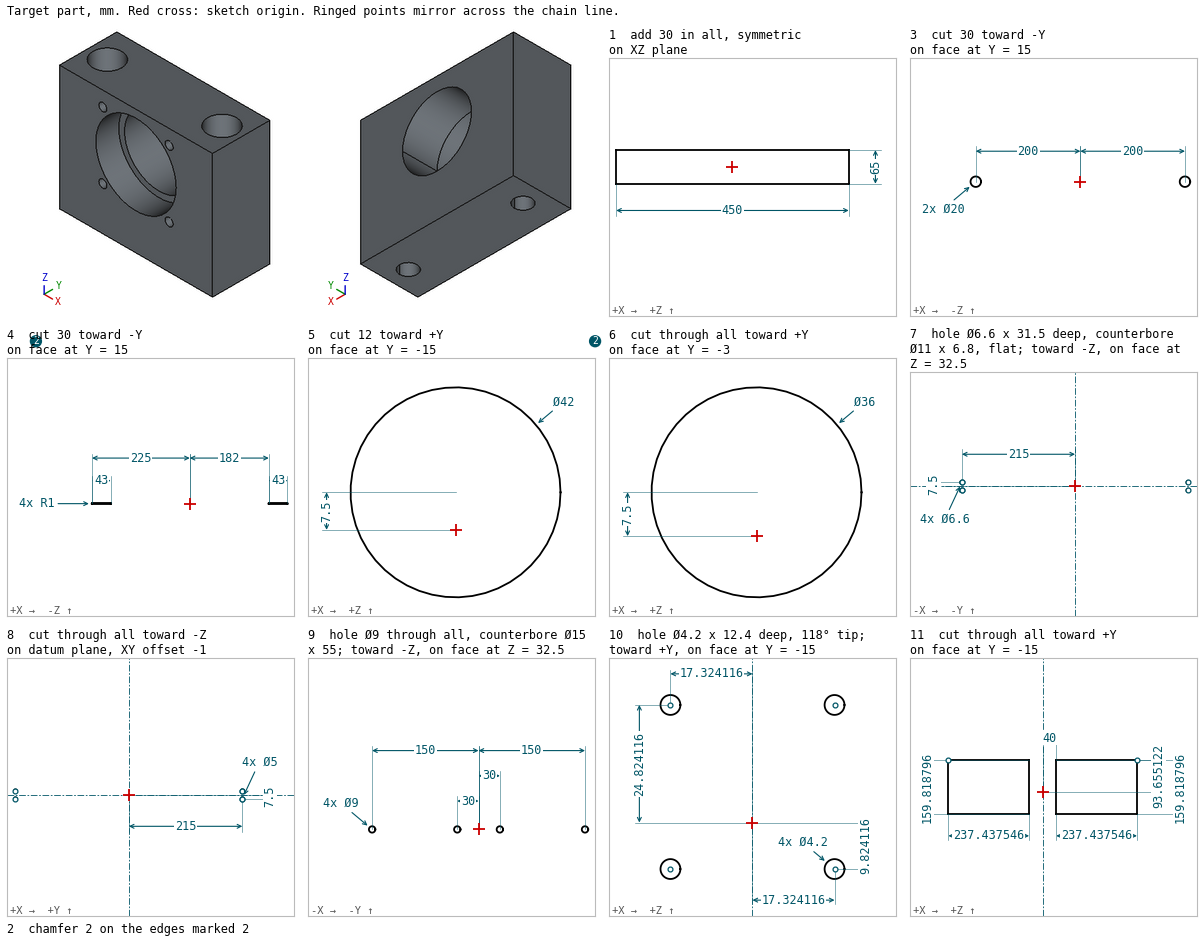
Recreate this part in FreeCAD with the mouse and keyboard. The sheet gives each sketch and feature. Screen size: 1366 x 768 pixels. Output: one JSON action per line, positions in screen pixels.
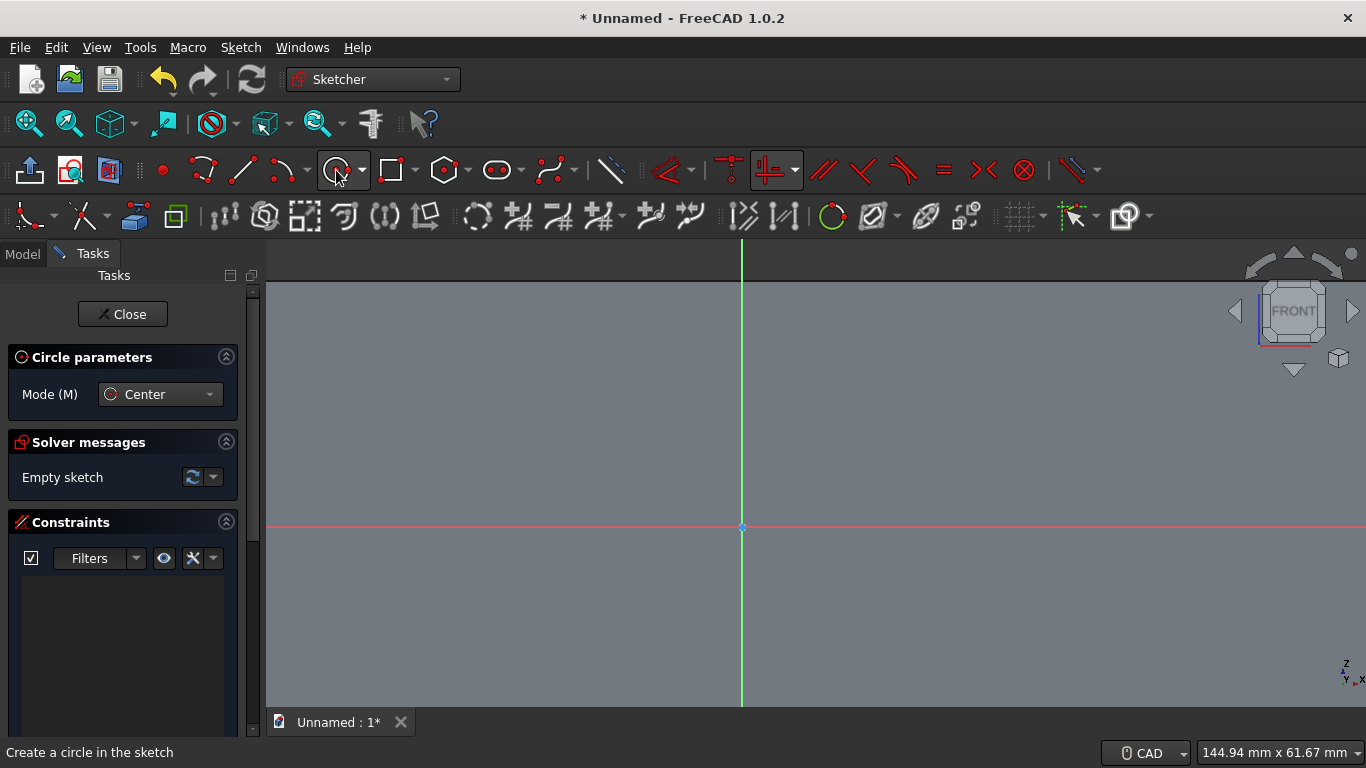
{"action": "left_click", "coordinate": [742, 471]}
{"action": "mouse_move", "coordinate": [855, 358]}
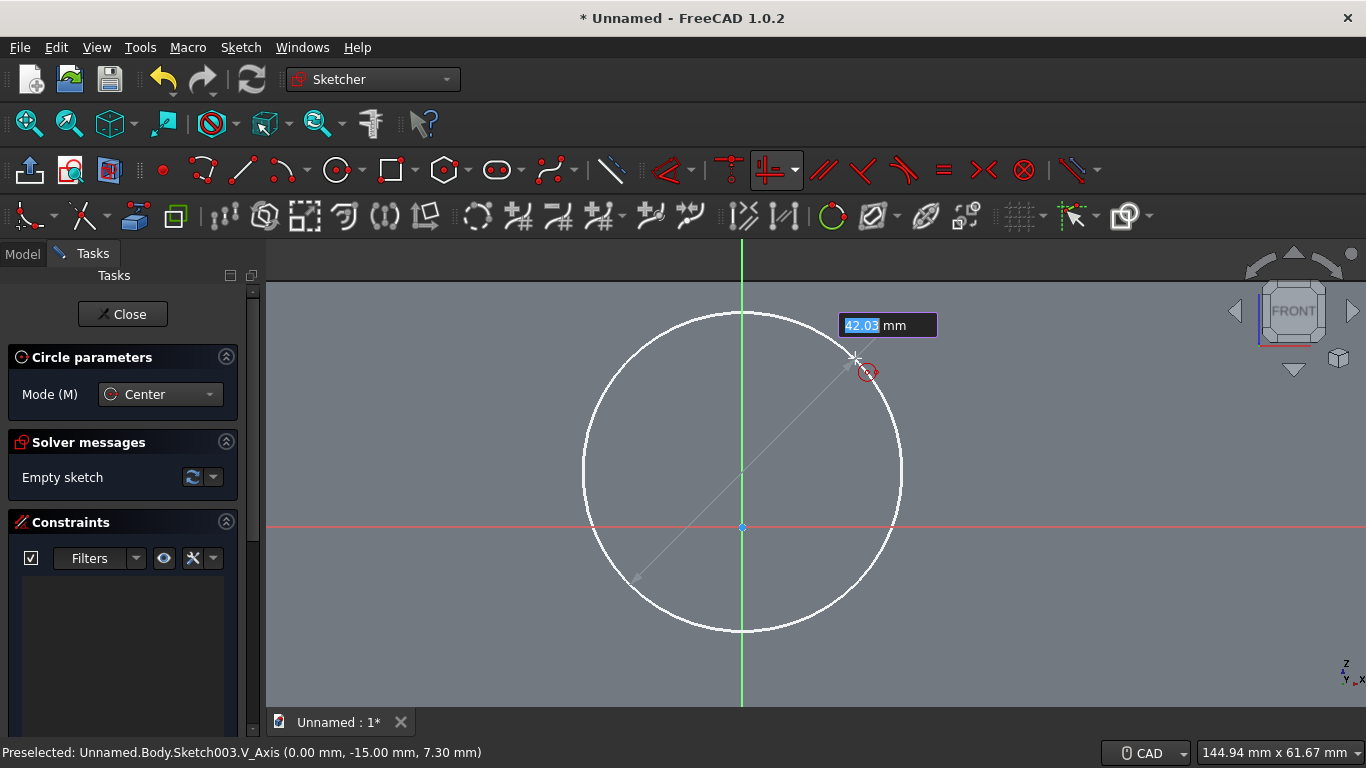
{"action": "type", "text": "42"}
{"action": "key", "text": "Return"}
{"action": "key", "text": "Escape"}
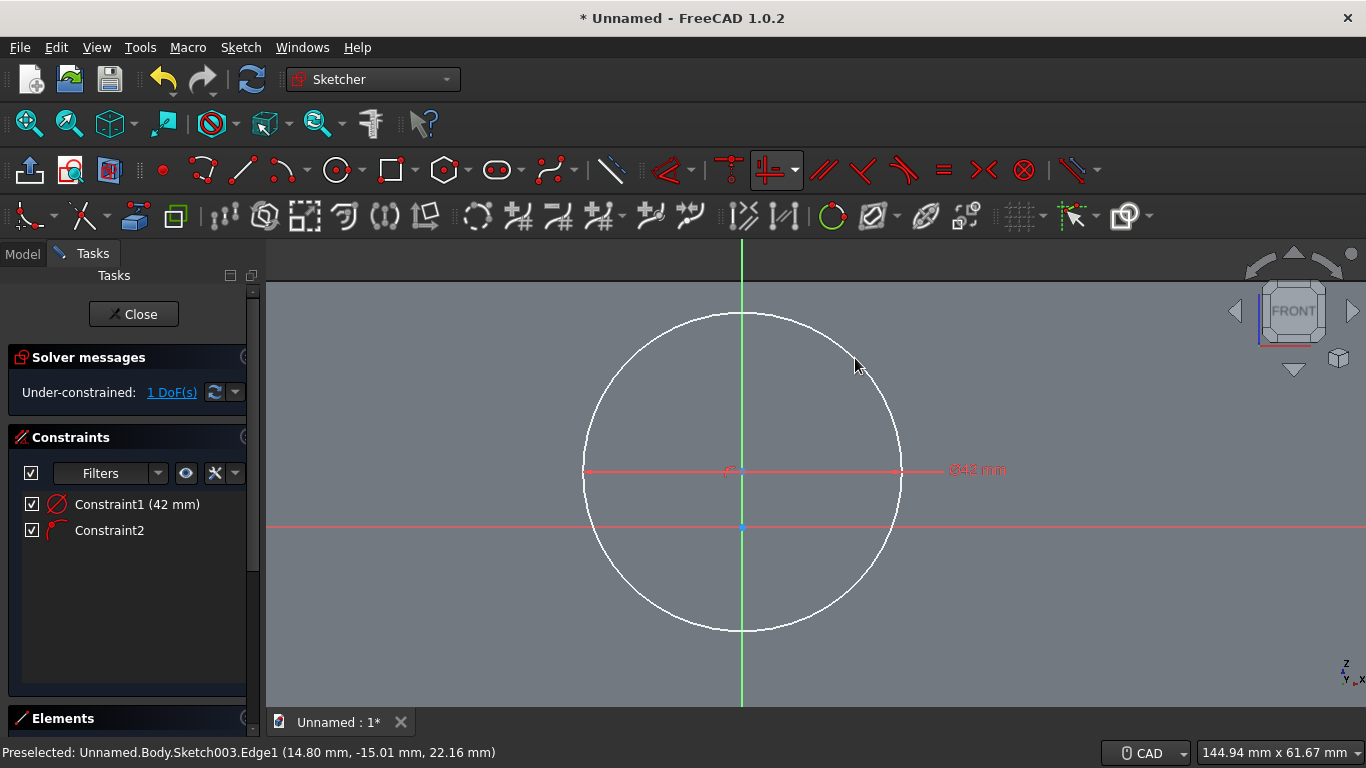
{"action": "key", "text": "d"}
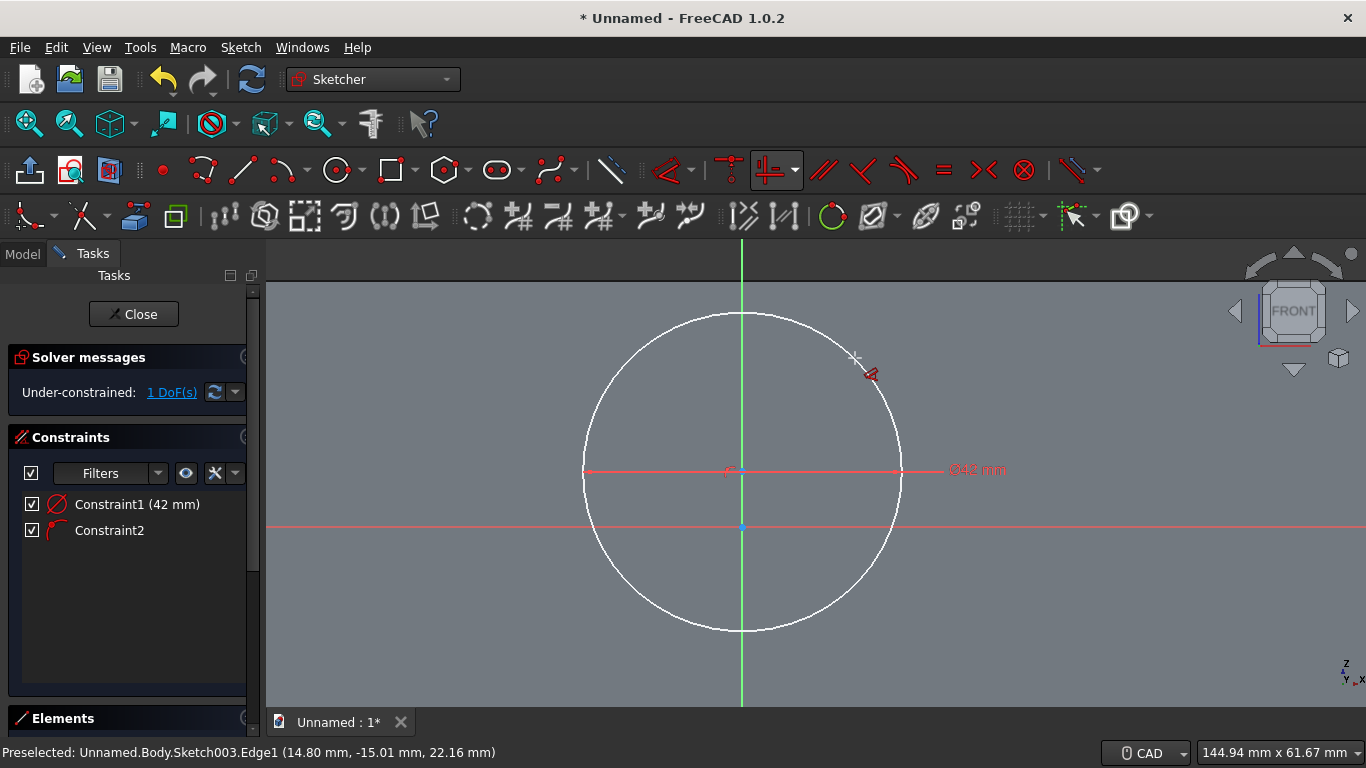
{"action": "left_click", "coordinate": [742, 472]}
{"action": "left_click", "coordinate": [776, 500]}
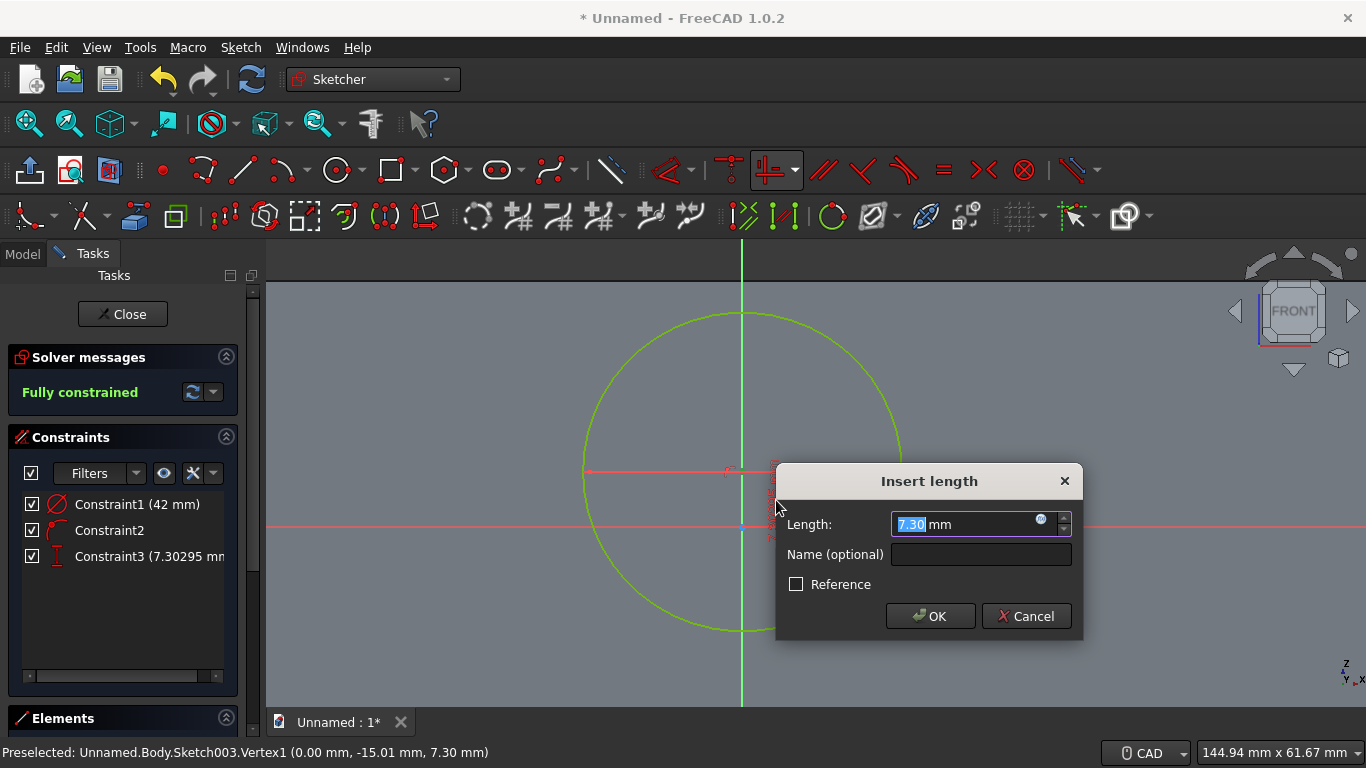
{"action": "type", "text": "7.5"}
{"action": "key", "text": "Return"}
{"action": "key", "text": "Escape"}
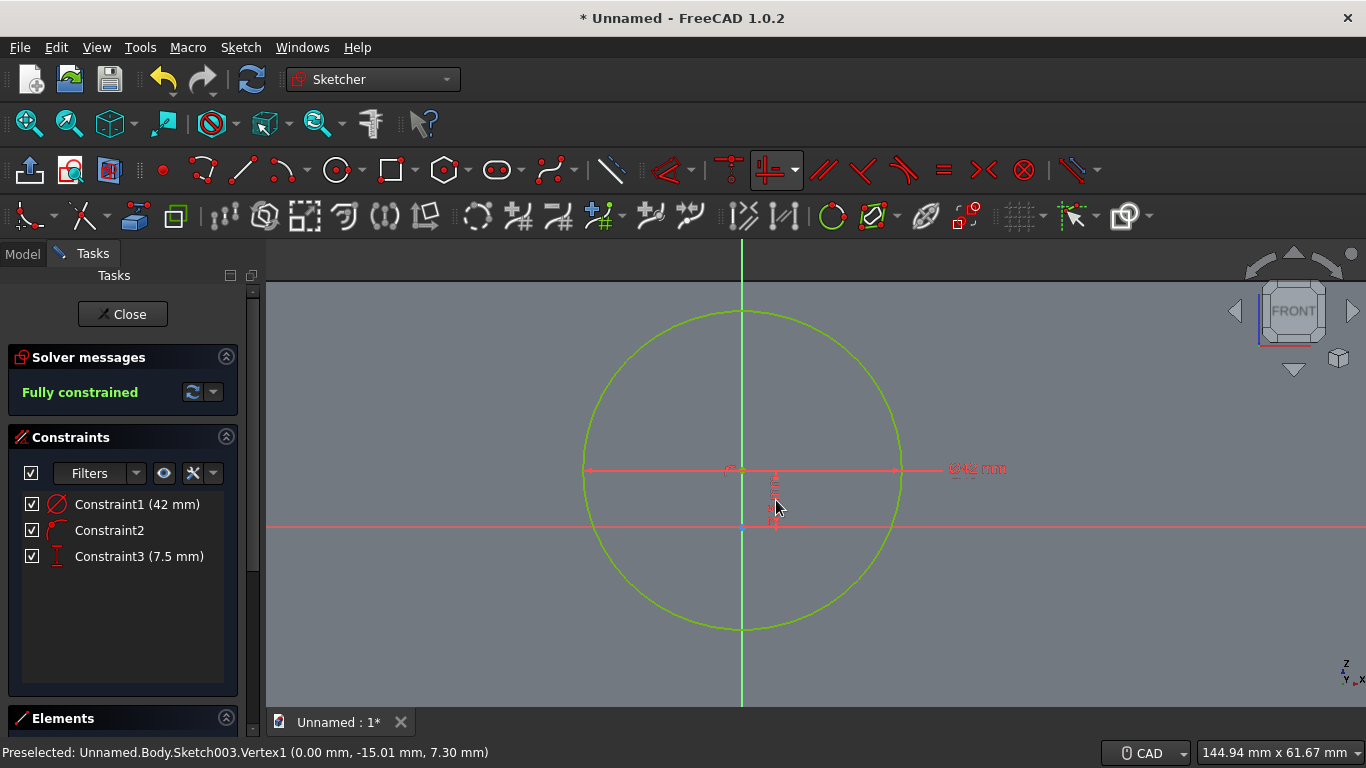
{"action": "left_click", "coordinate": [123, 314]}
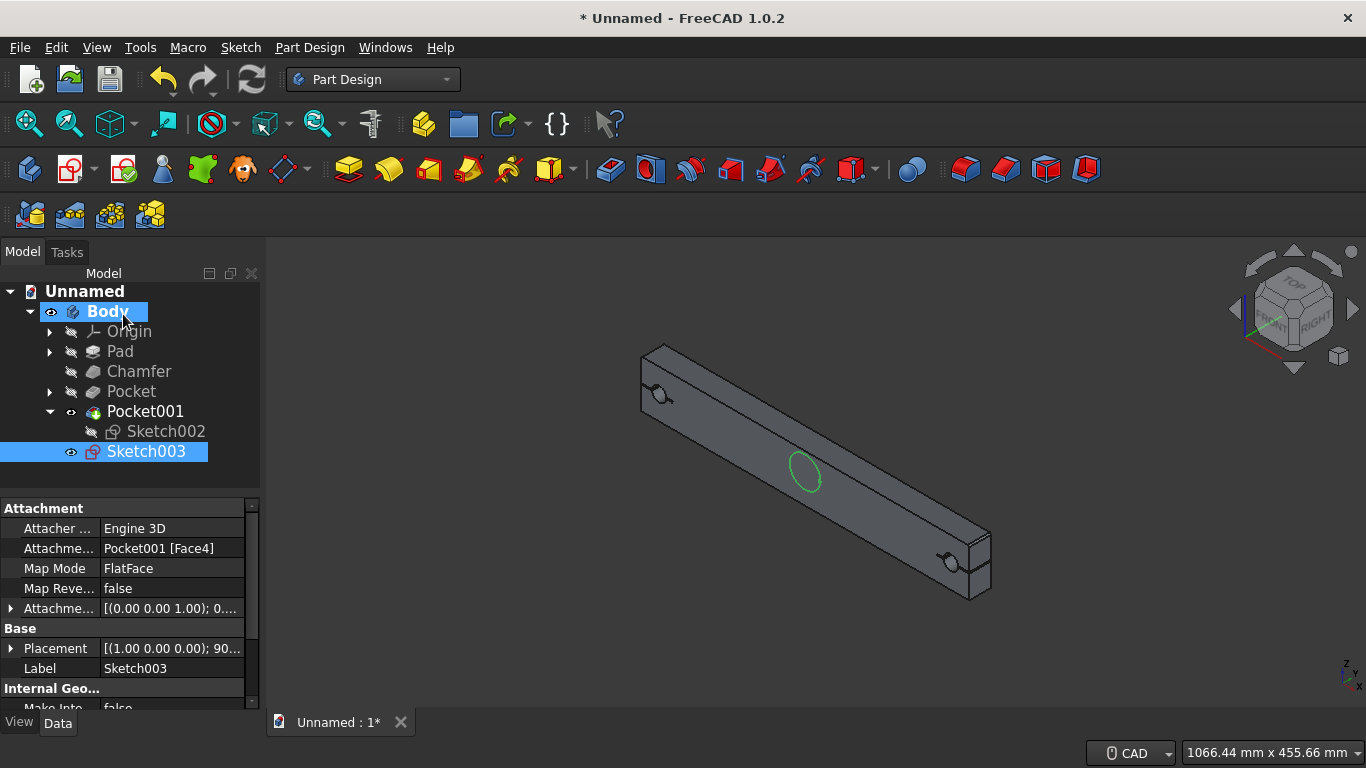
{"action": "left_click", "coordinate": [612, 170]}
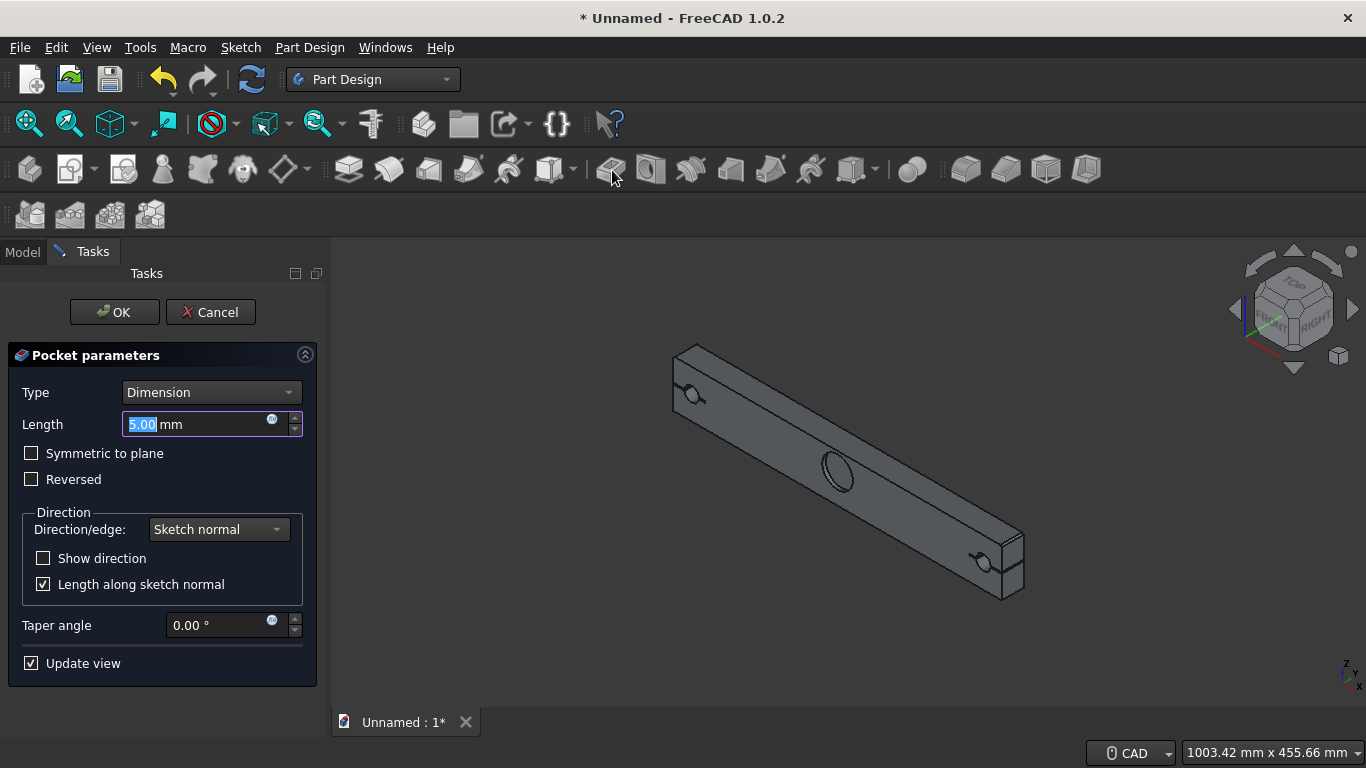
{"action": "type", "text": "12"}
{"action": "key", "text": "Tab"}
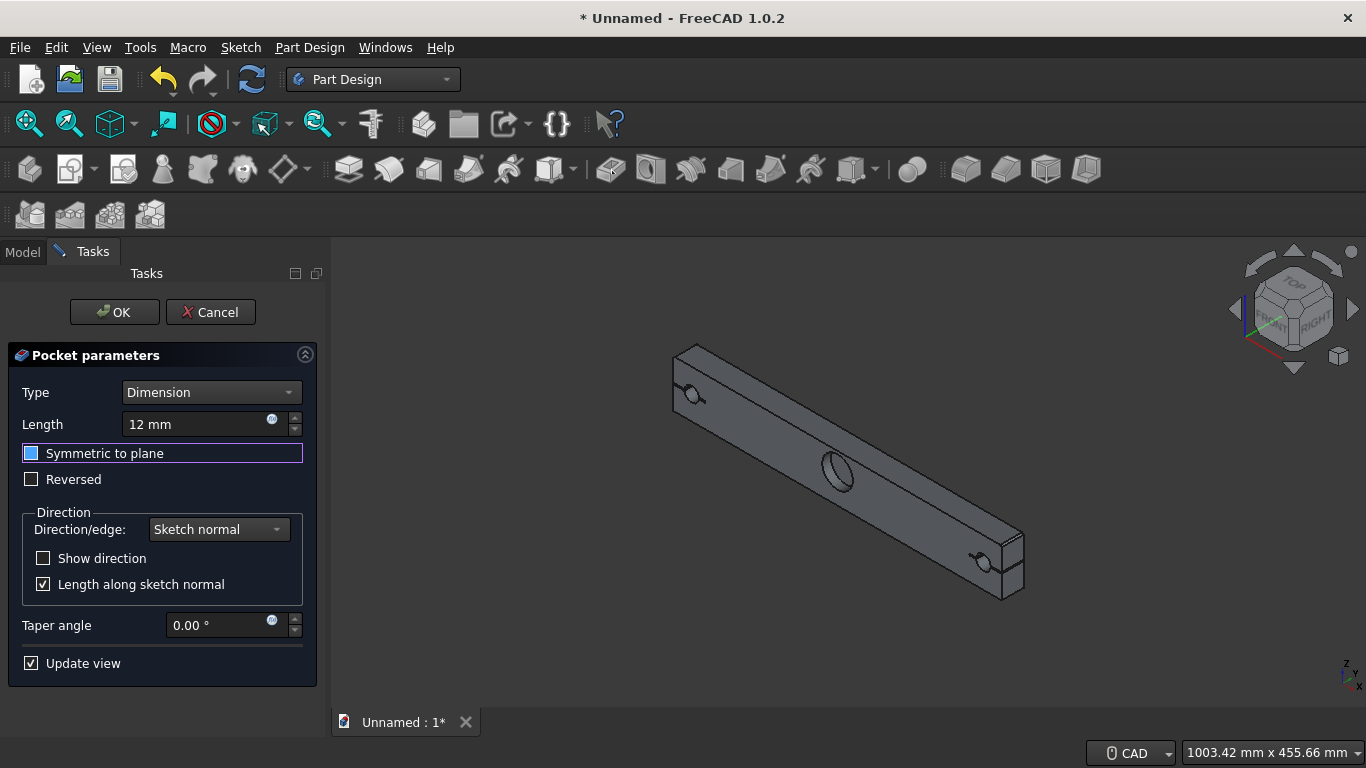
{"action": "left_click", "coordinate": [115, 312]}